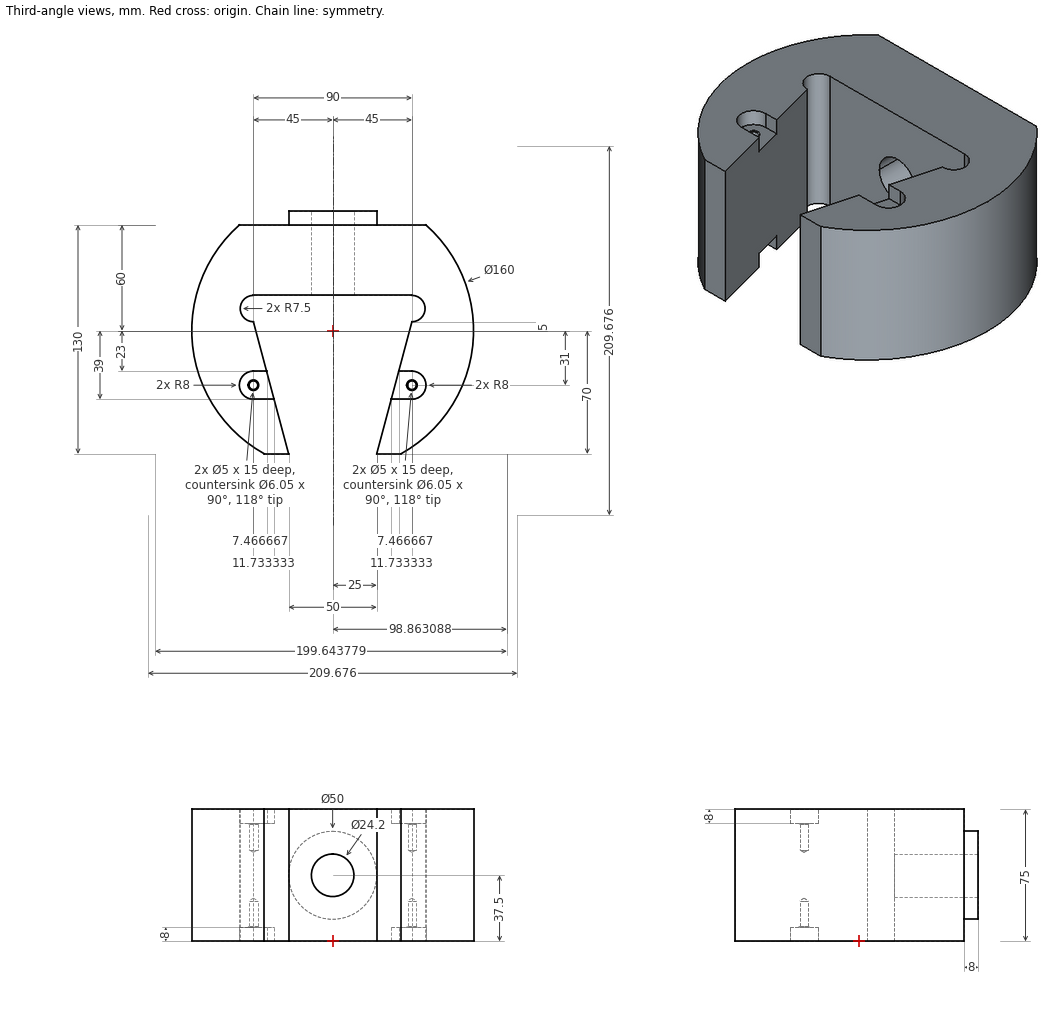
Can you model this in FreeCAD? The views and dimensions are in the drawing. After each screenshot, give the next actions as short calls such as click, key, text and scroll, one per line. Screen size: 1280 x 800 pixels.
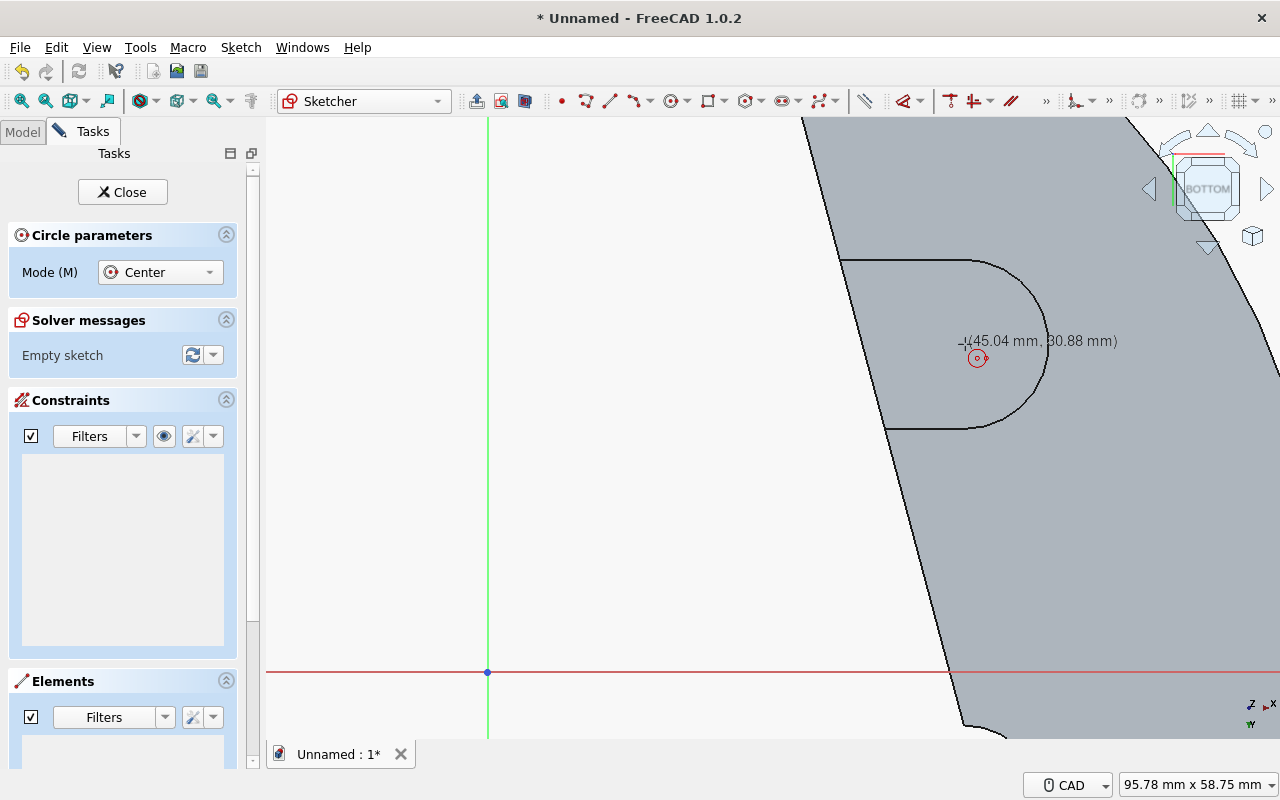
click(964, 344)
move(983, 326)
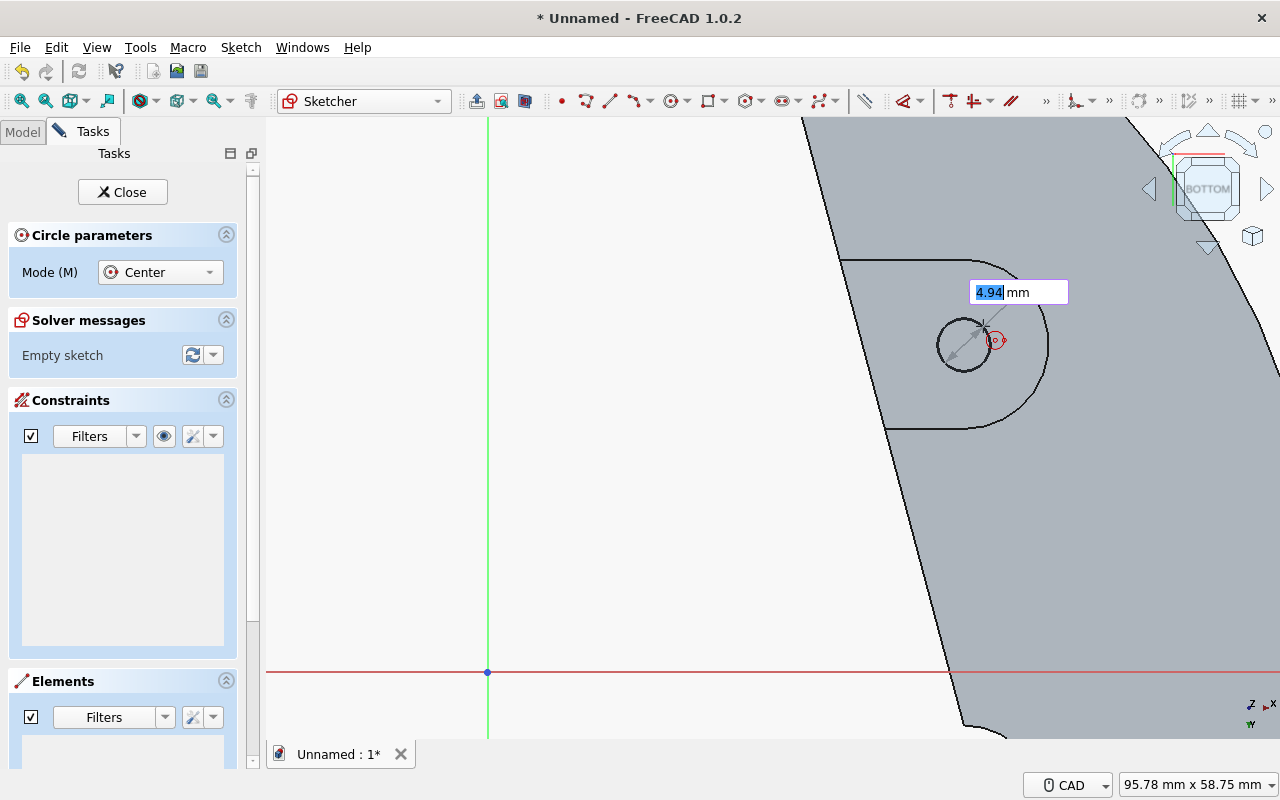
text(5)
key(Return)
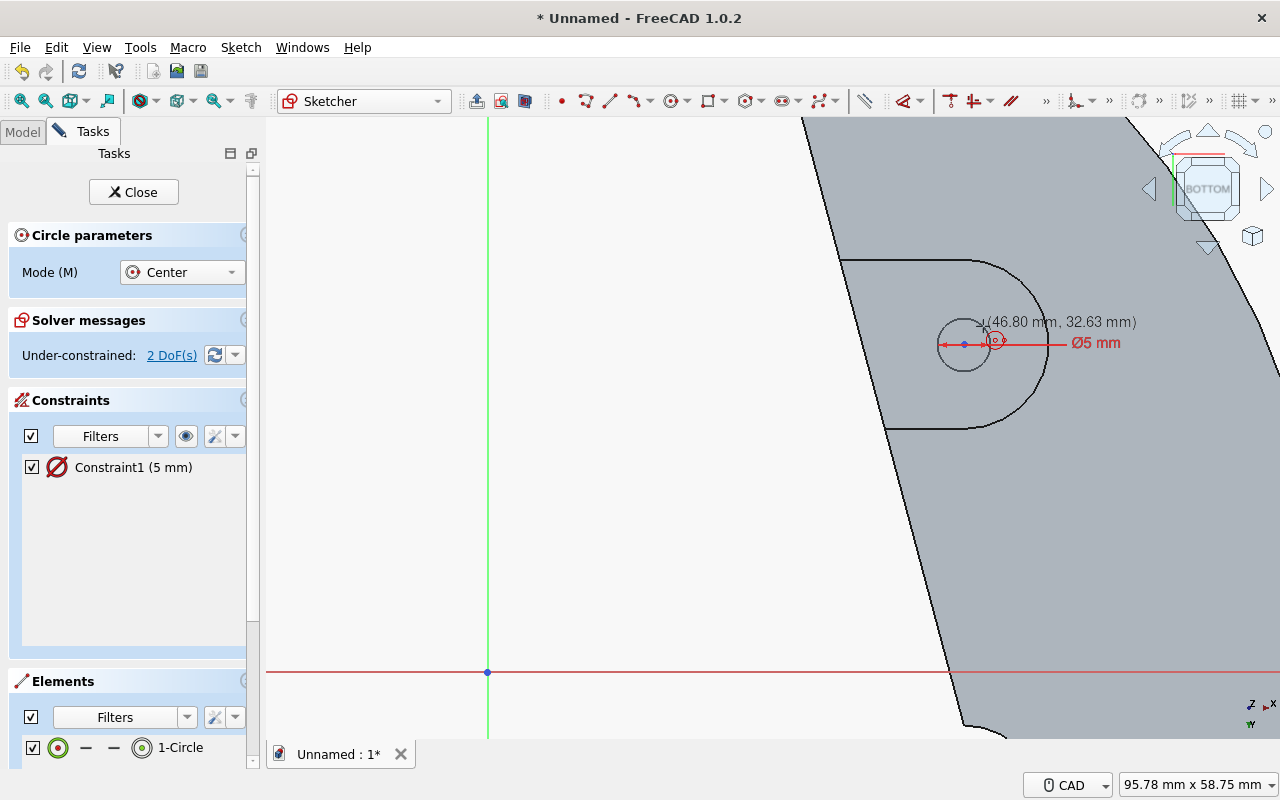
scroll(968, 346, down, 3)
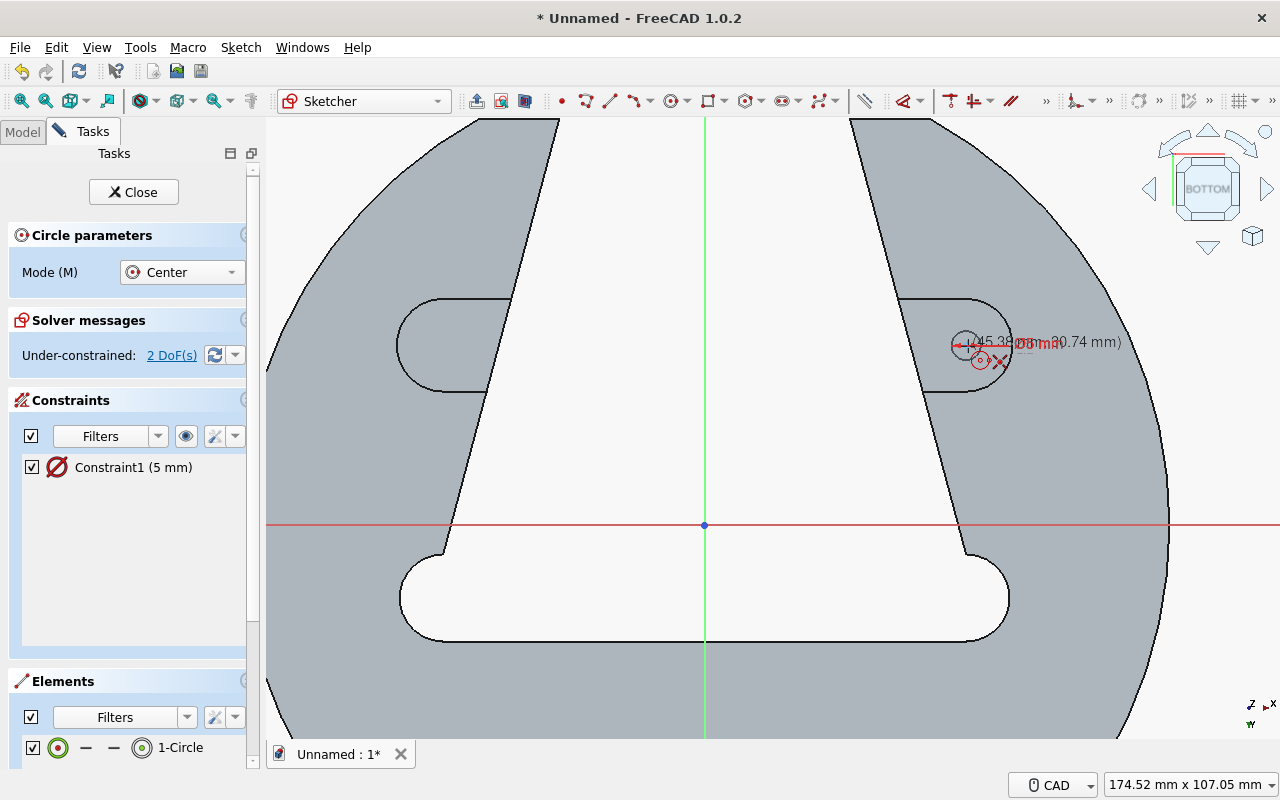
scroll(443, 345, up, 3)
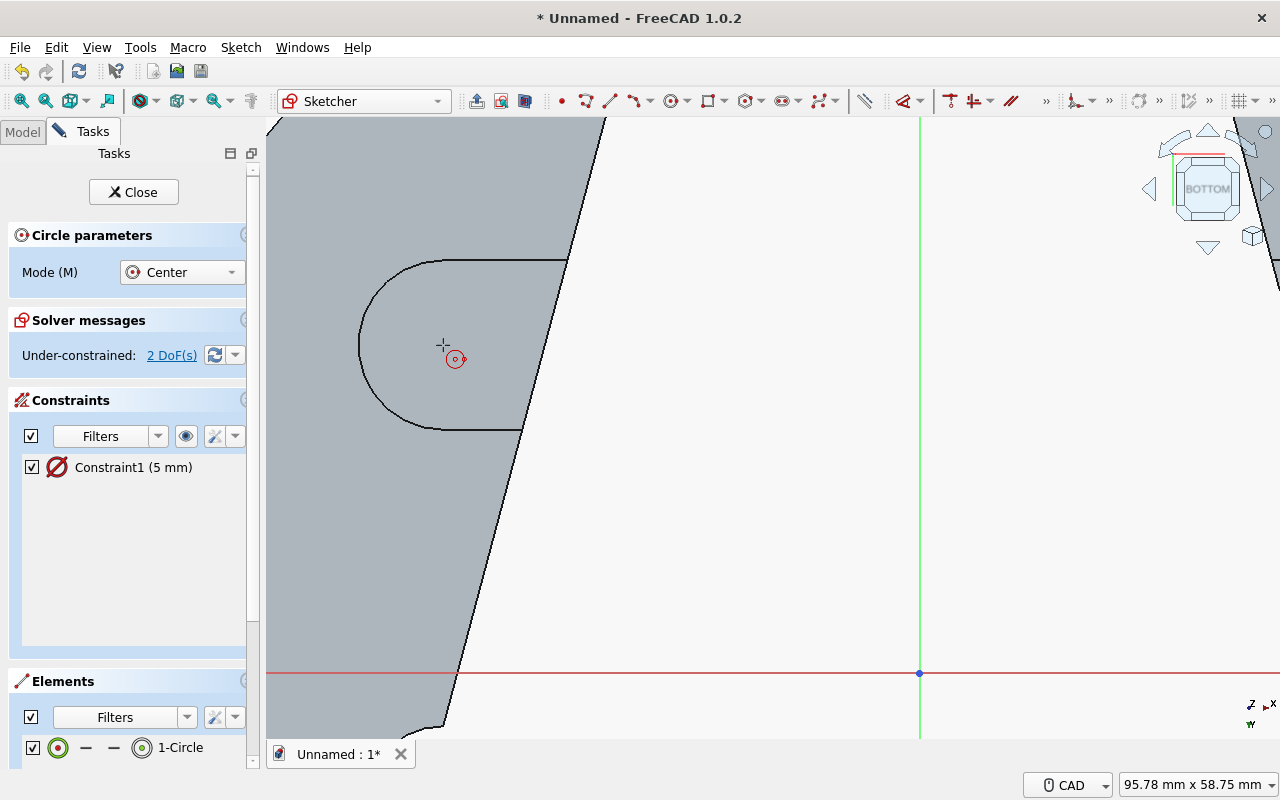
click(443, 345)
move(462, 326)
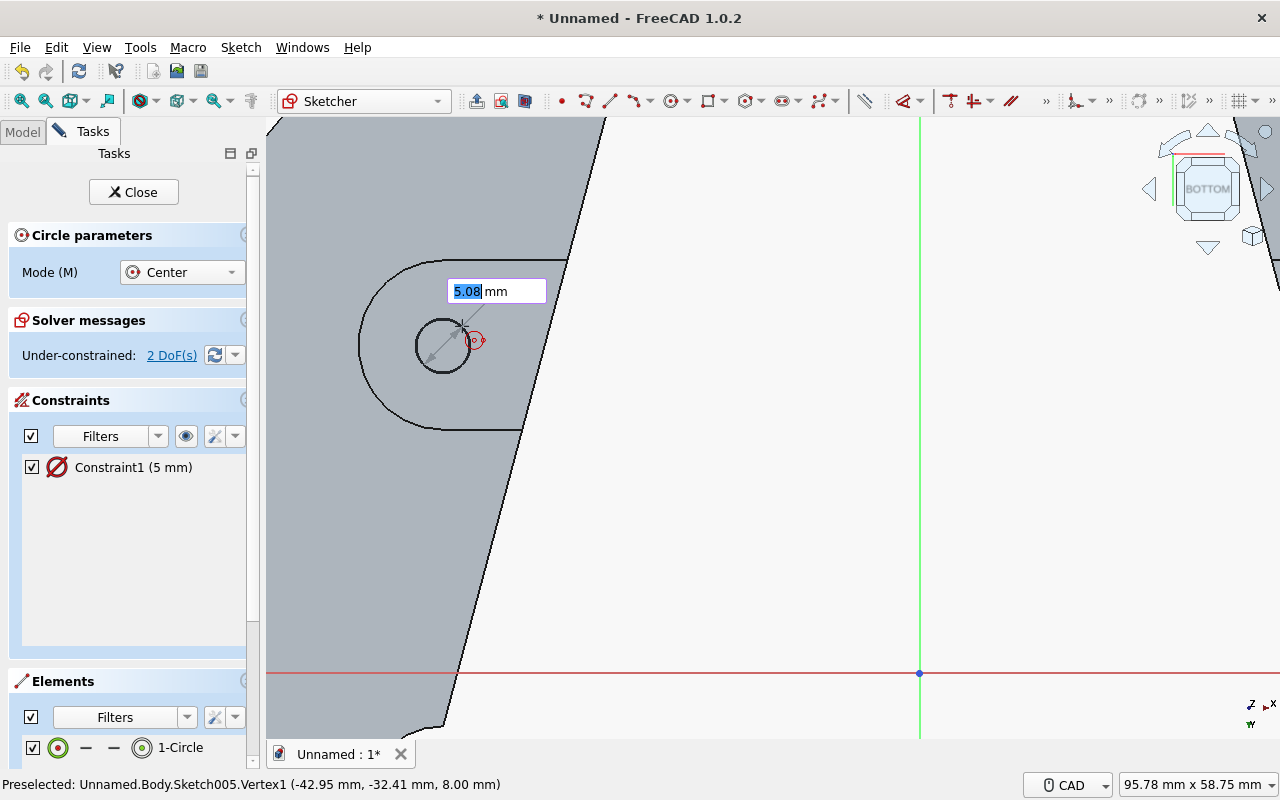
text(5)
key(Return)
key(Escape)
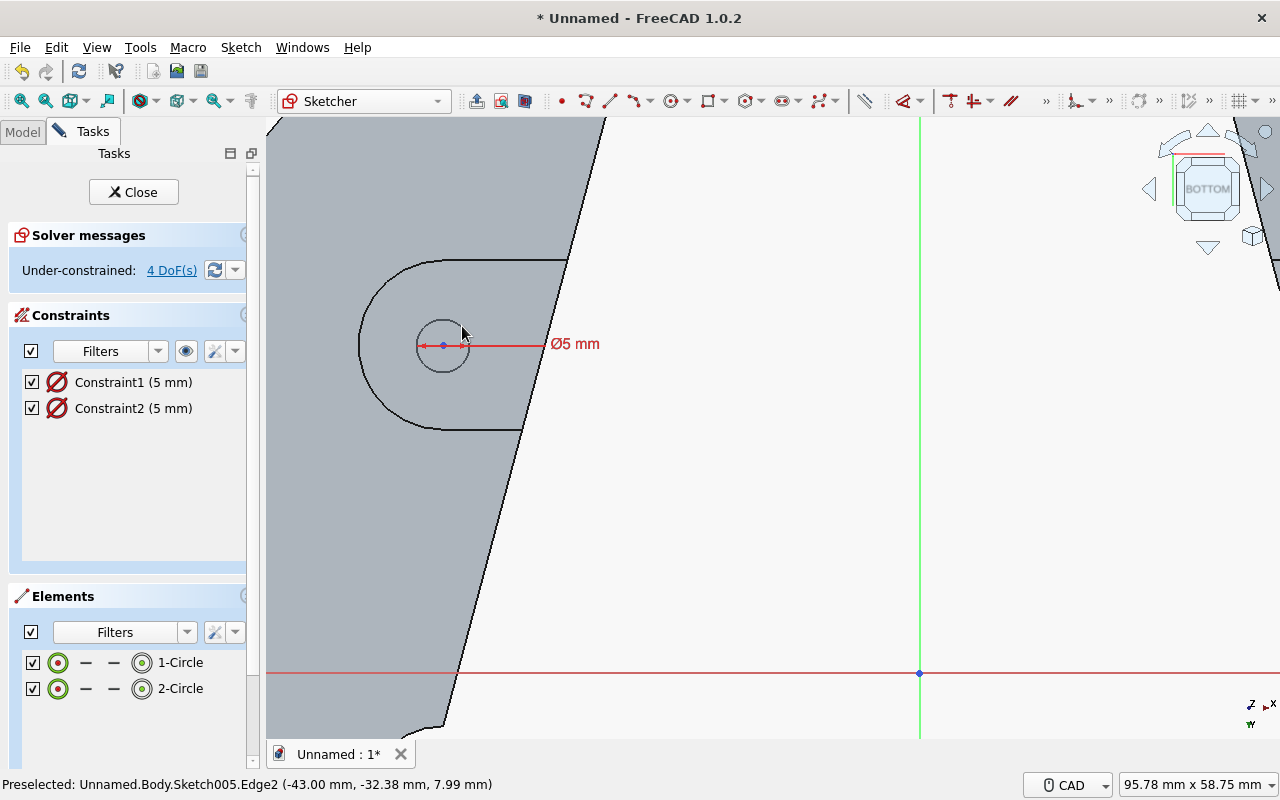
scroll(443, 345, down, 3)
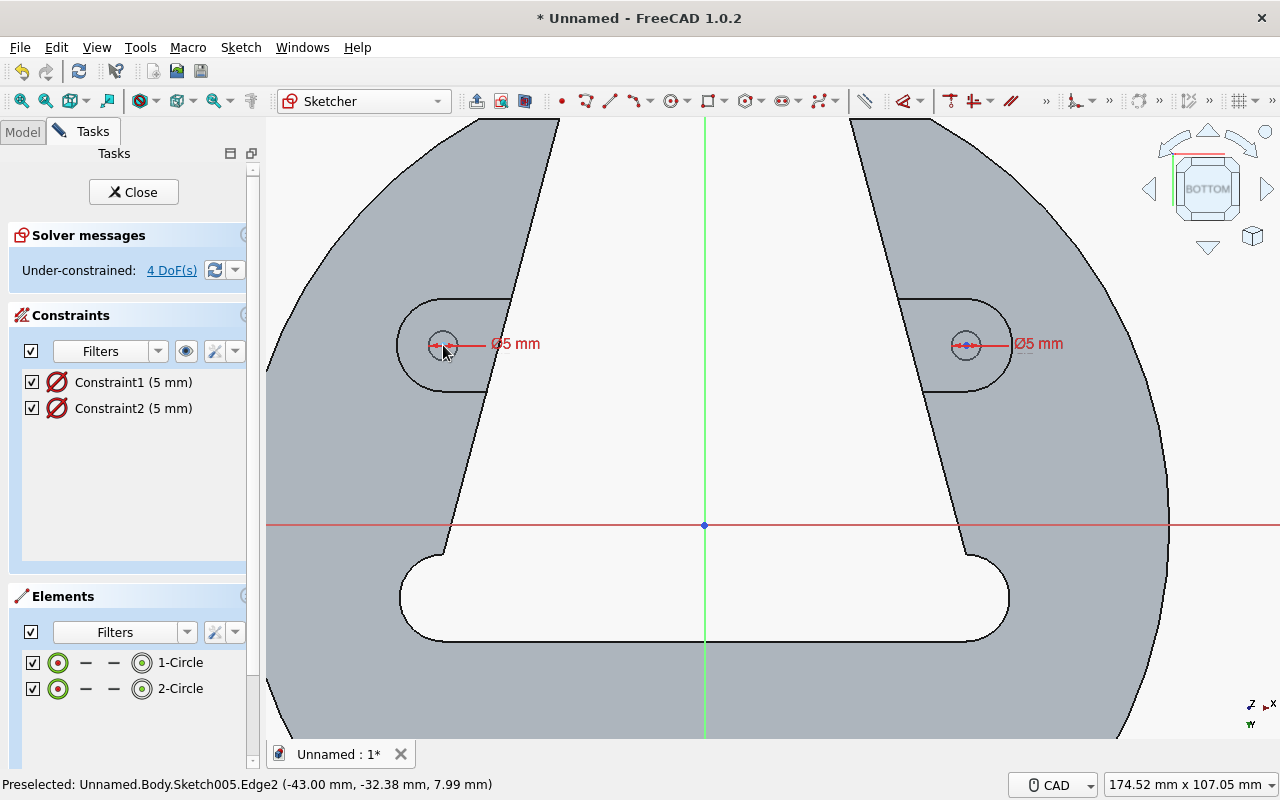
click(966, 346)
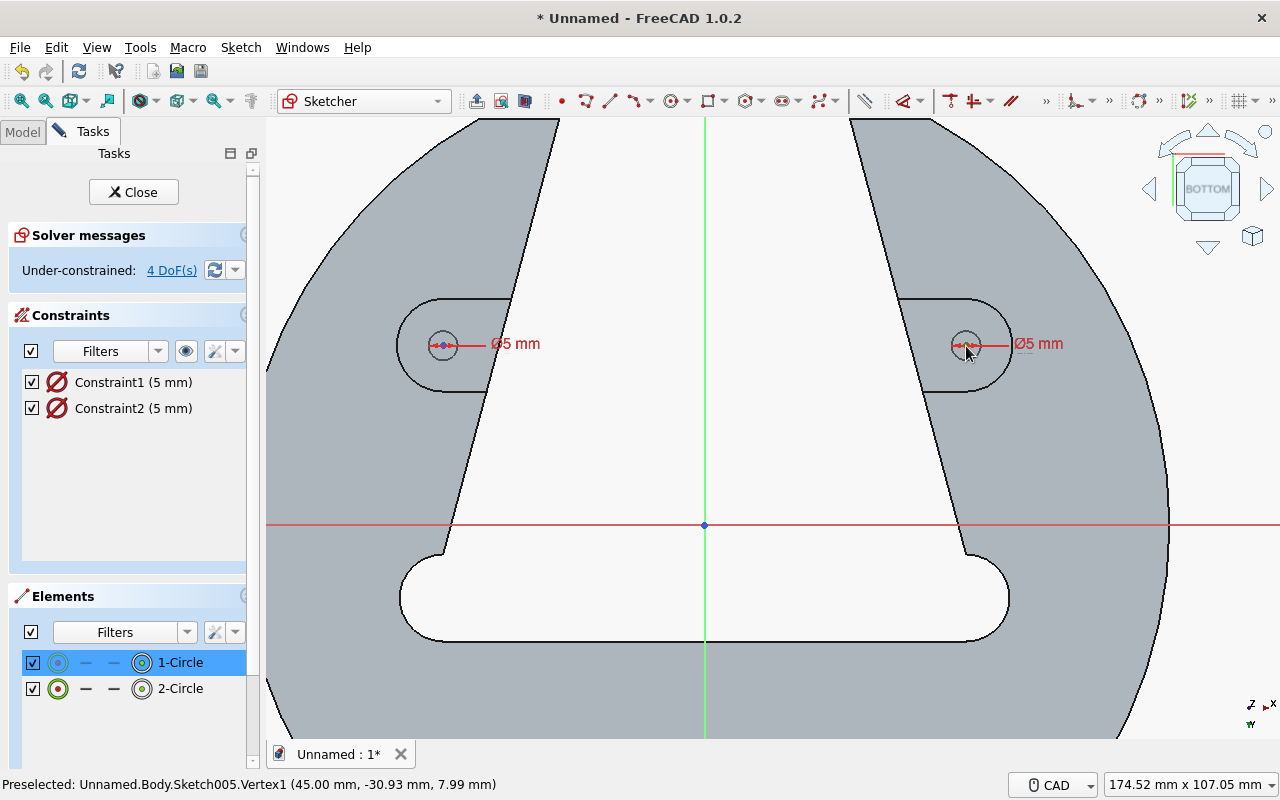
click(443, 346)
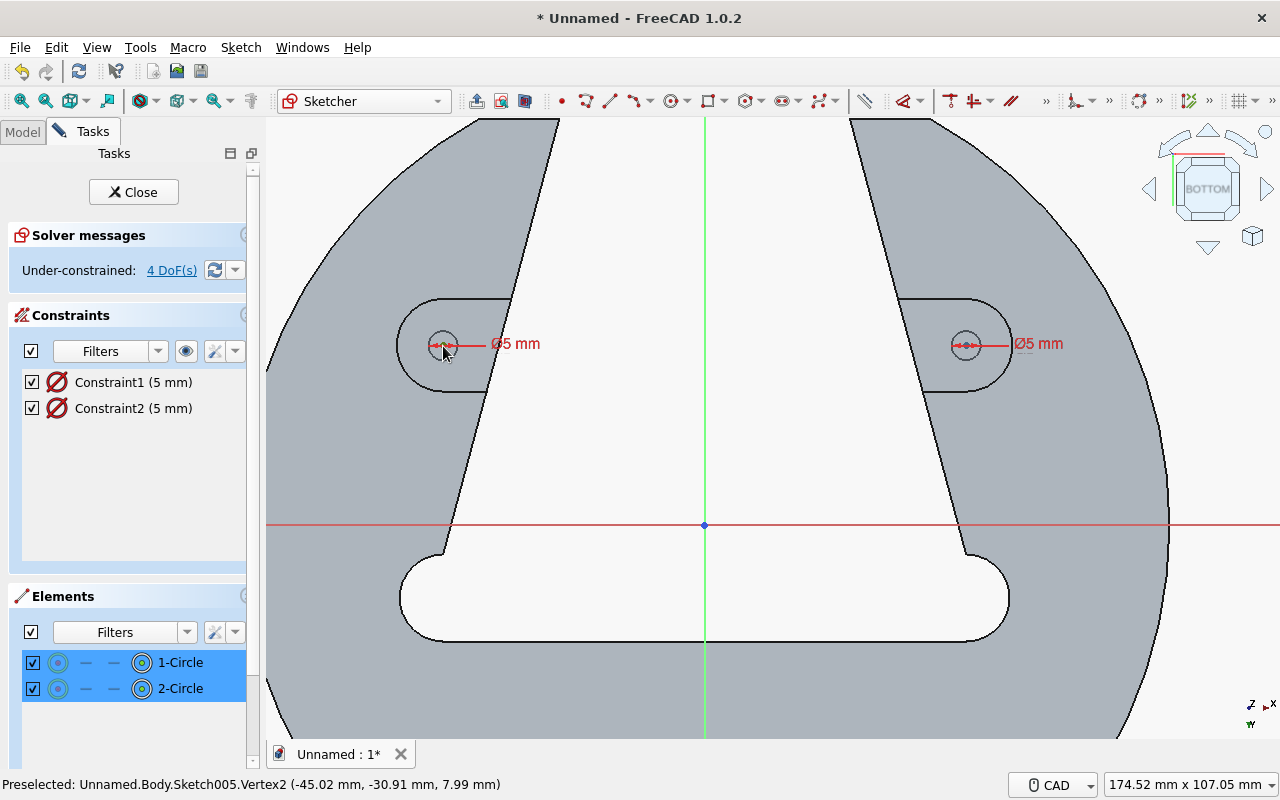
key(h)